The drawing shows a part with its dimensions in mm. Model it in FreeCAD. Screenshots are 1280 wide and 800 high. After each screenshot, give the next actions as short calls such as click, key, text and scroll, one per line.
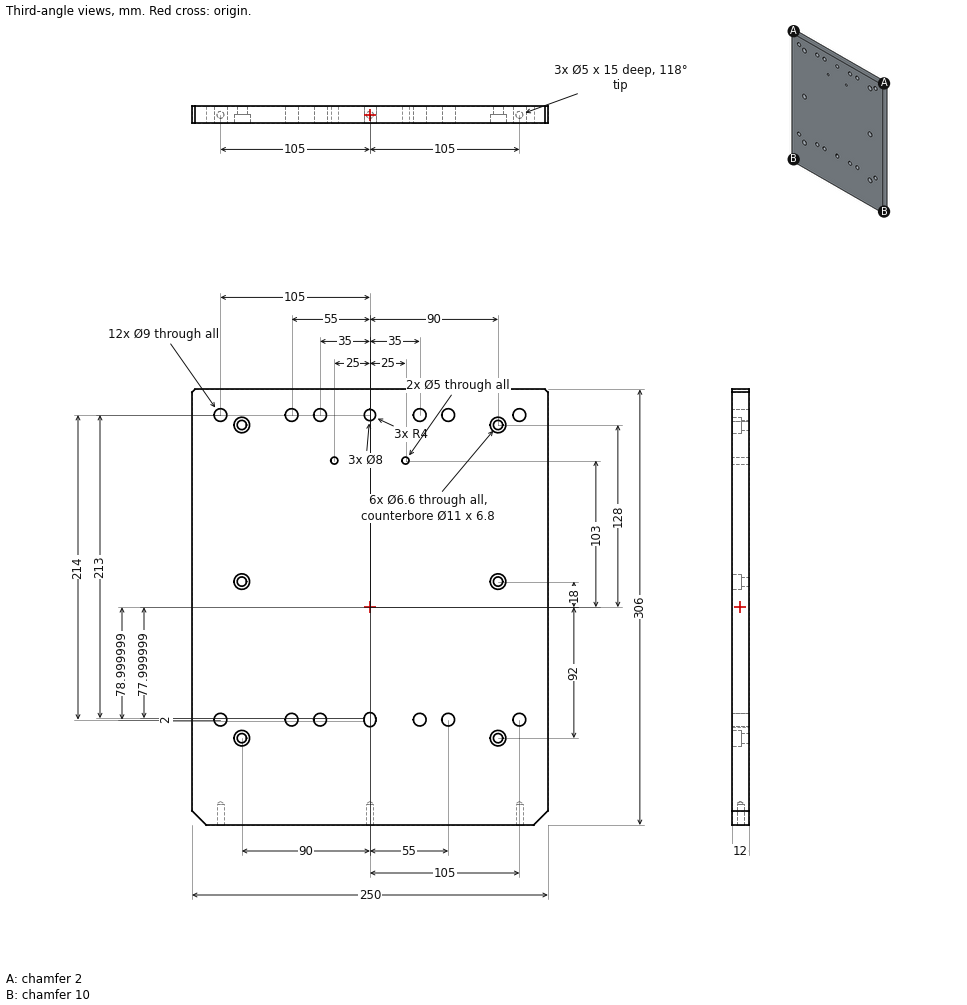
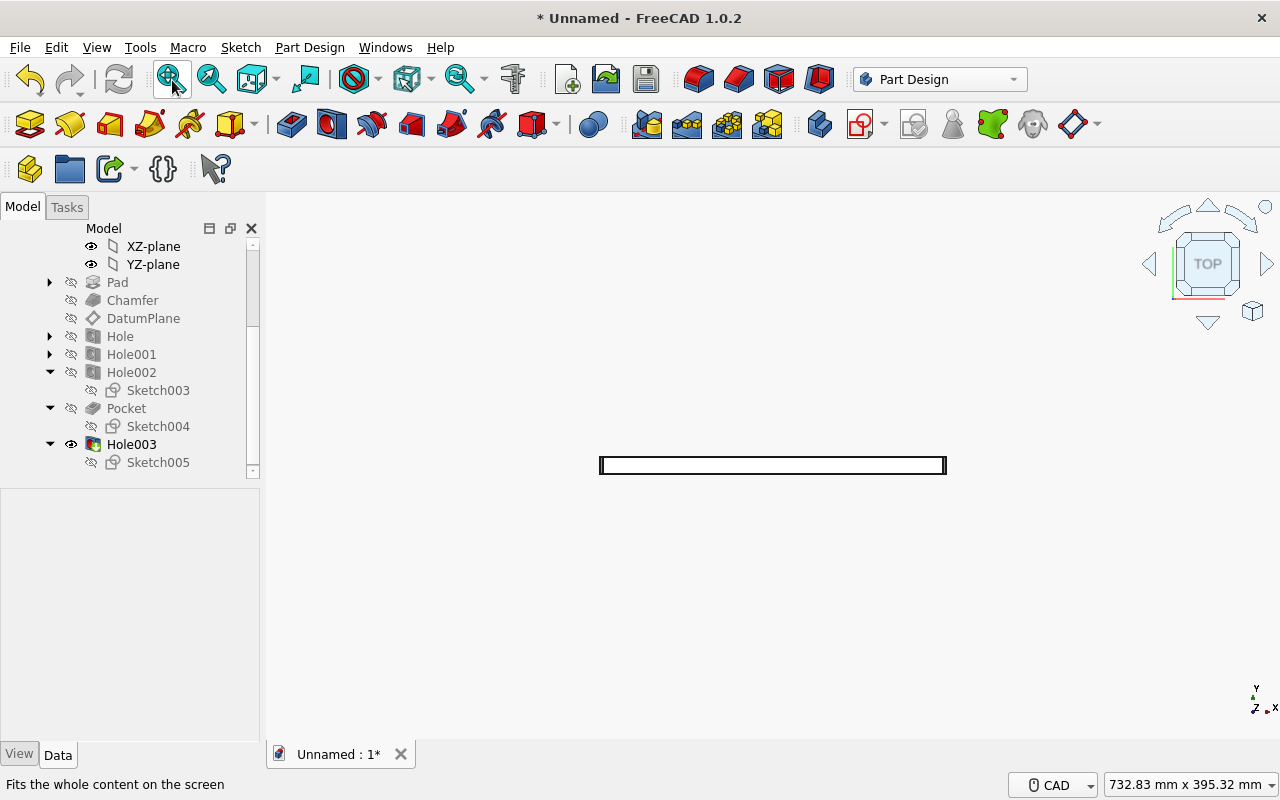
click(172, 80)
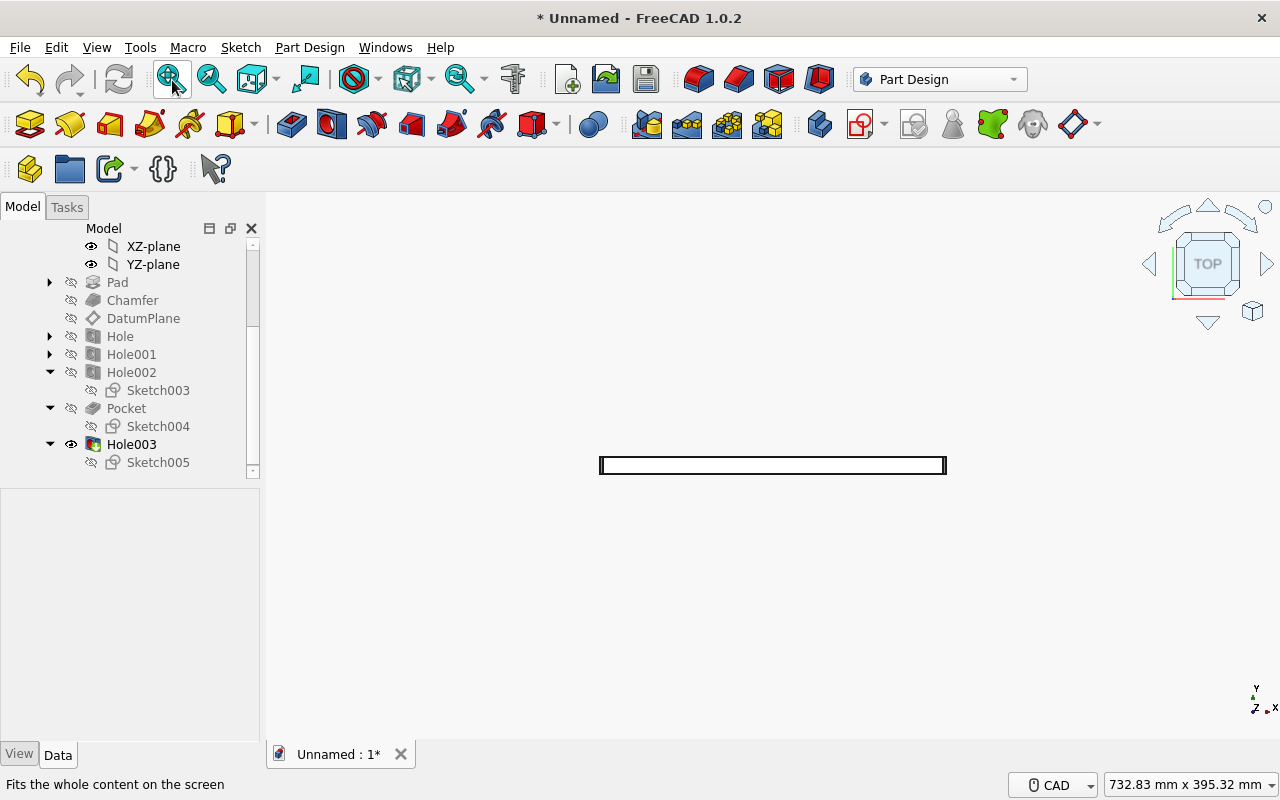
scroll(600, 464, up, 5)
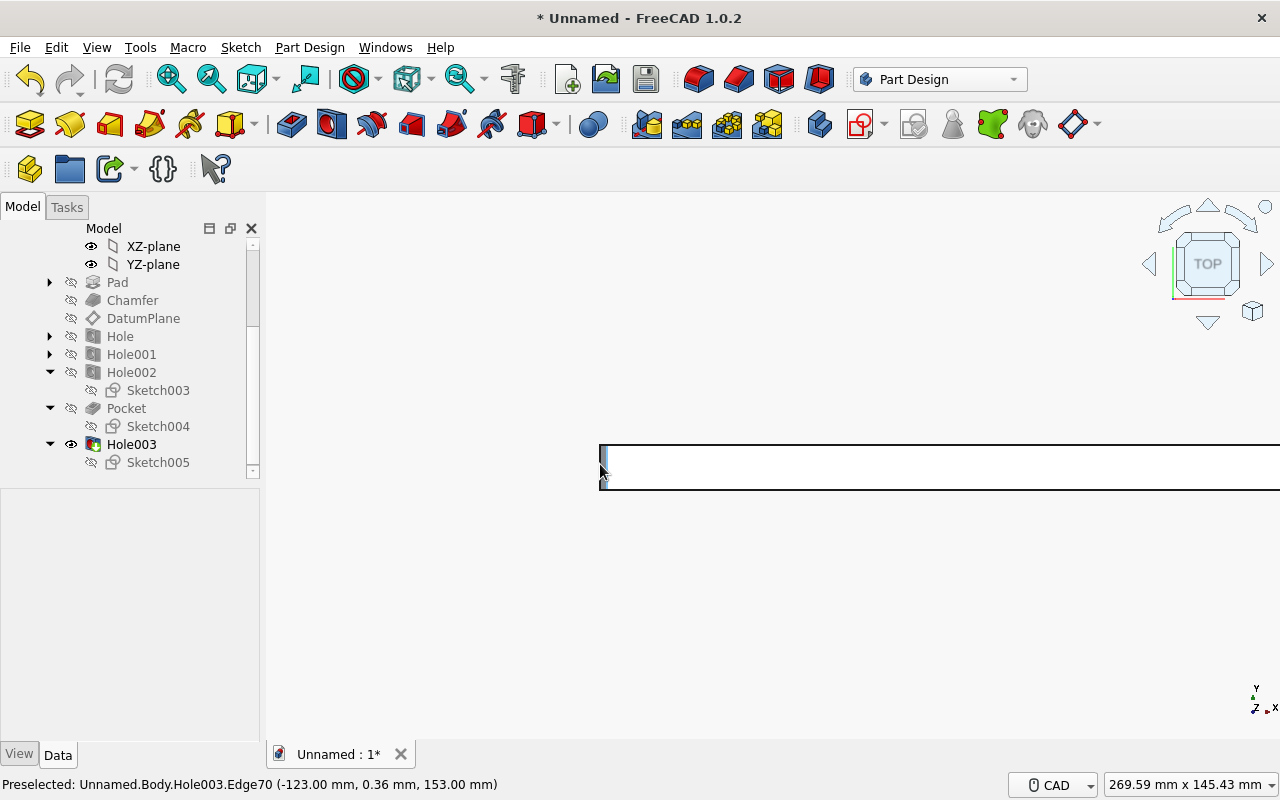
click(172, 80)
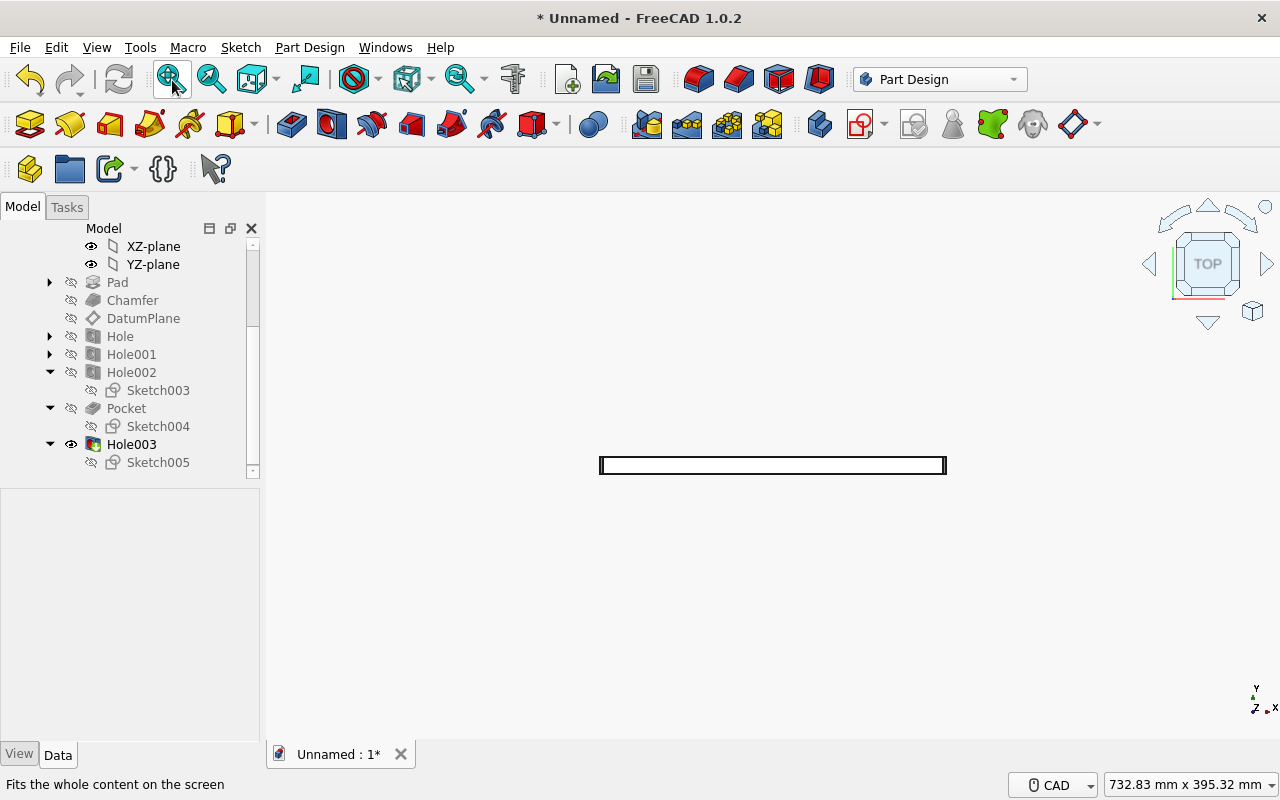
key(1)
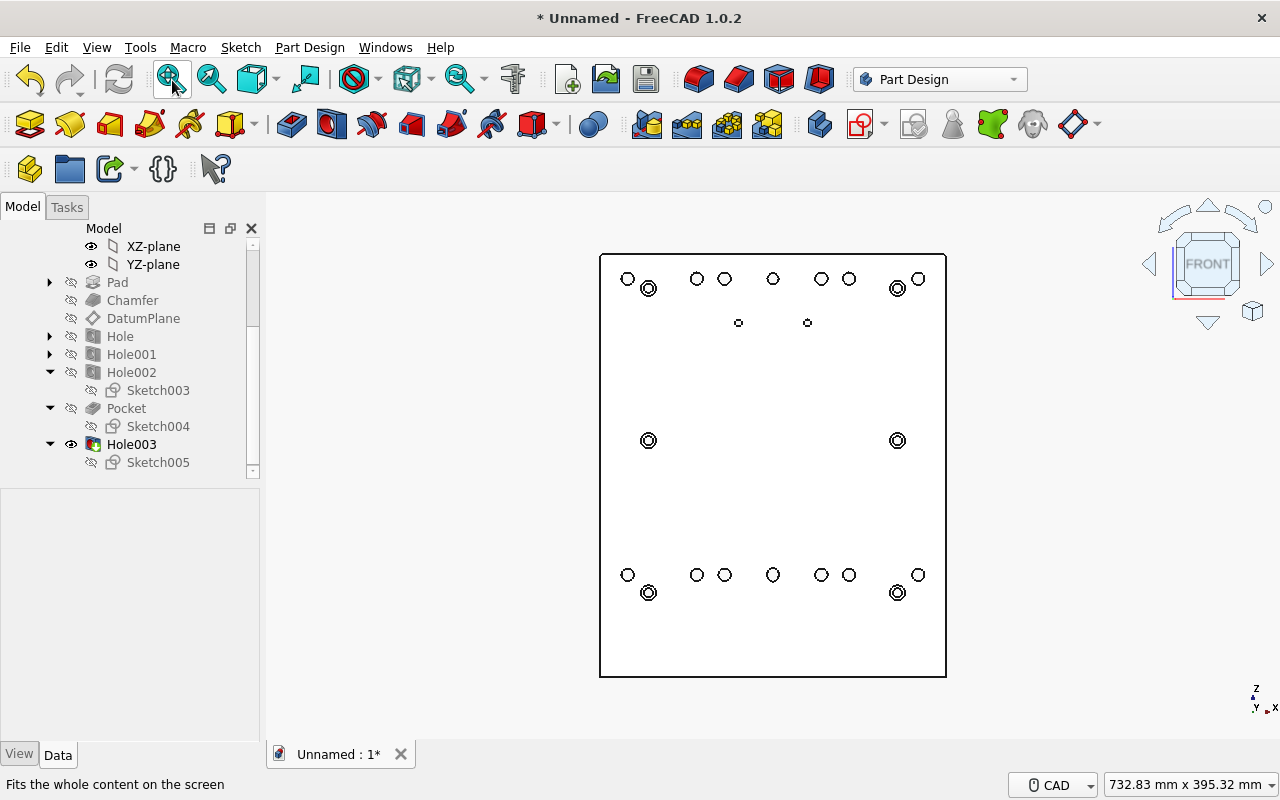
scroll(600, 676, up, 5)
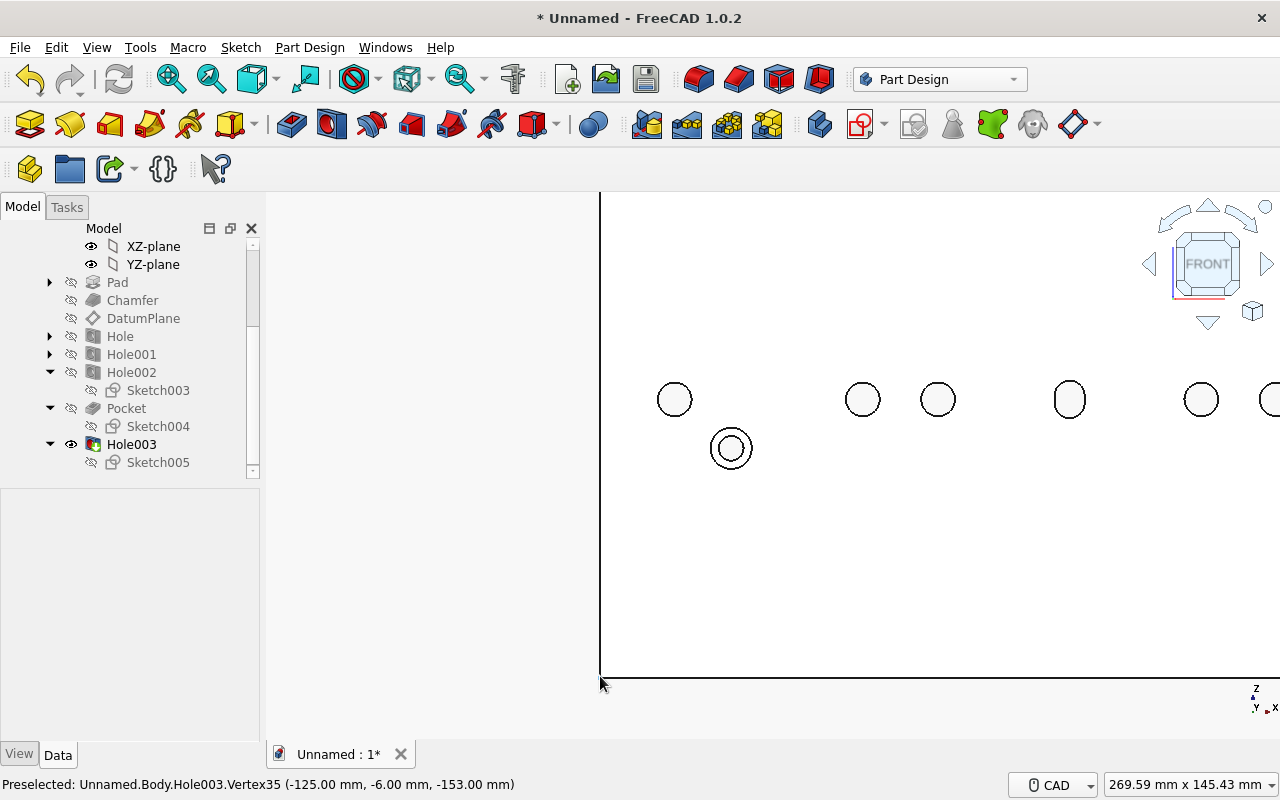
key(v)
key(f)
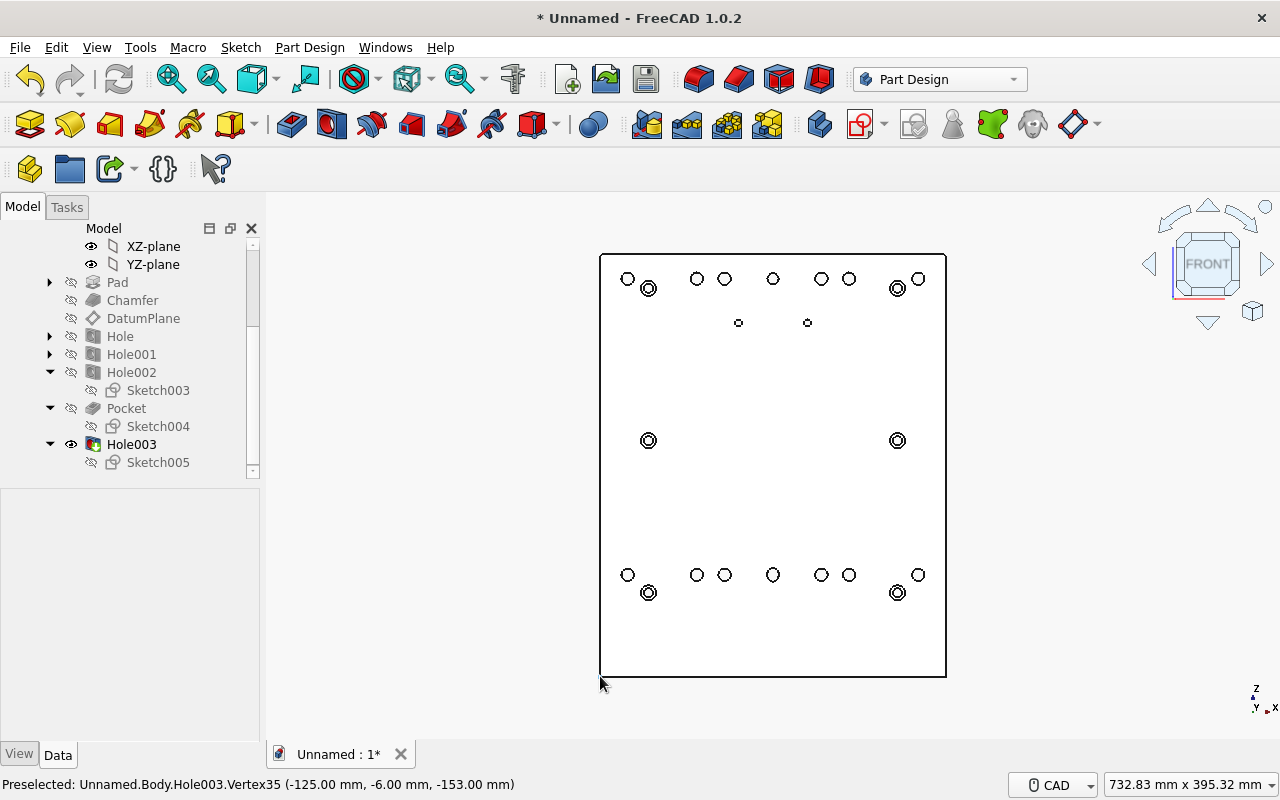
key(3)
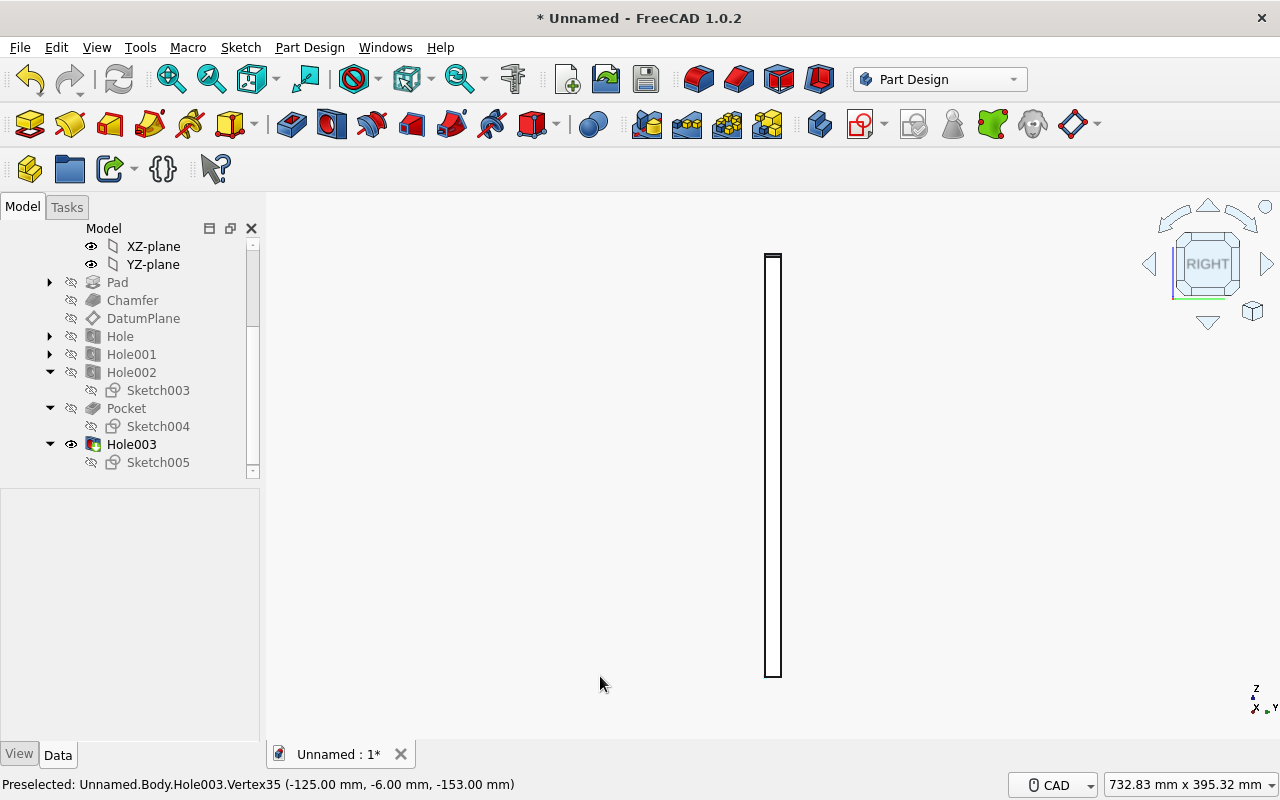
click(773, 676)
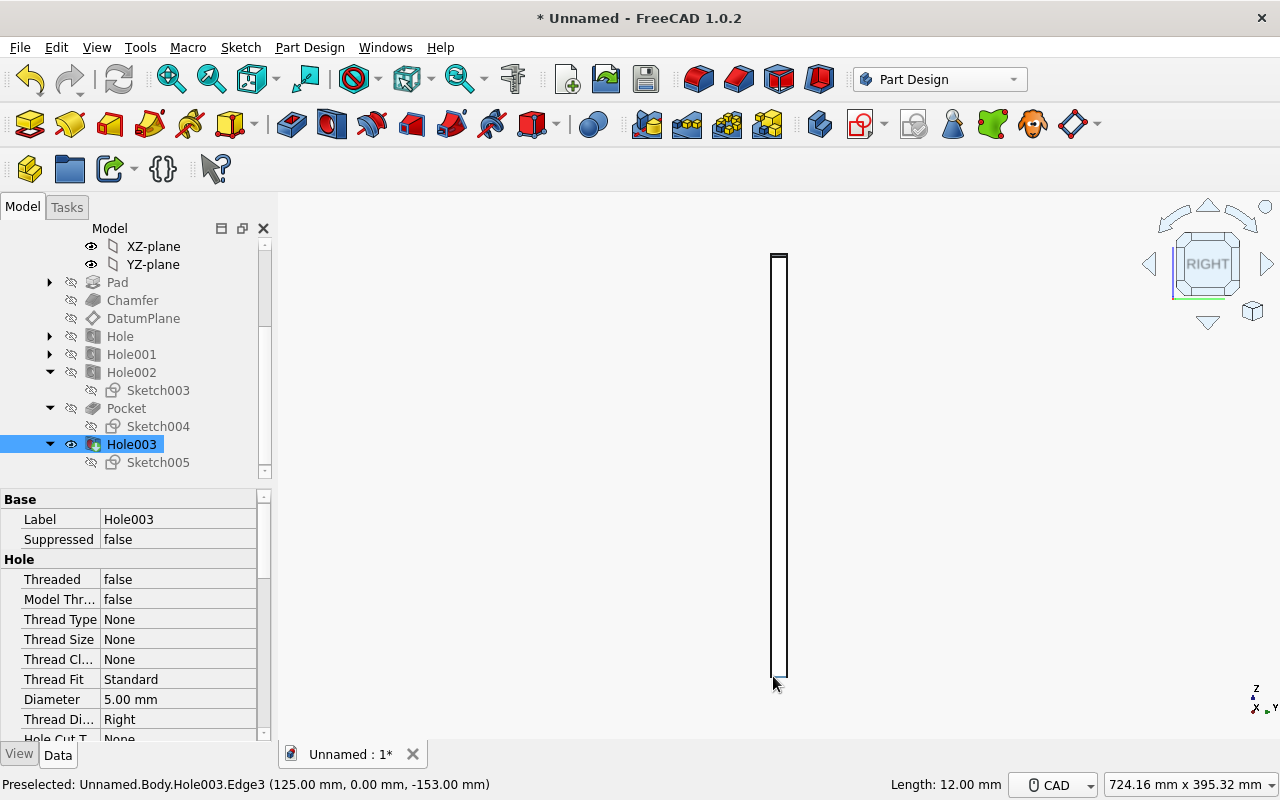
scroll(779, 676, up, 5)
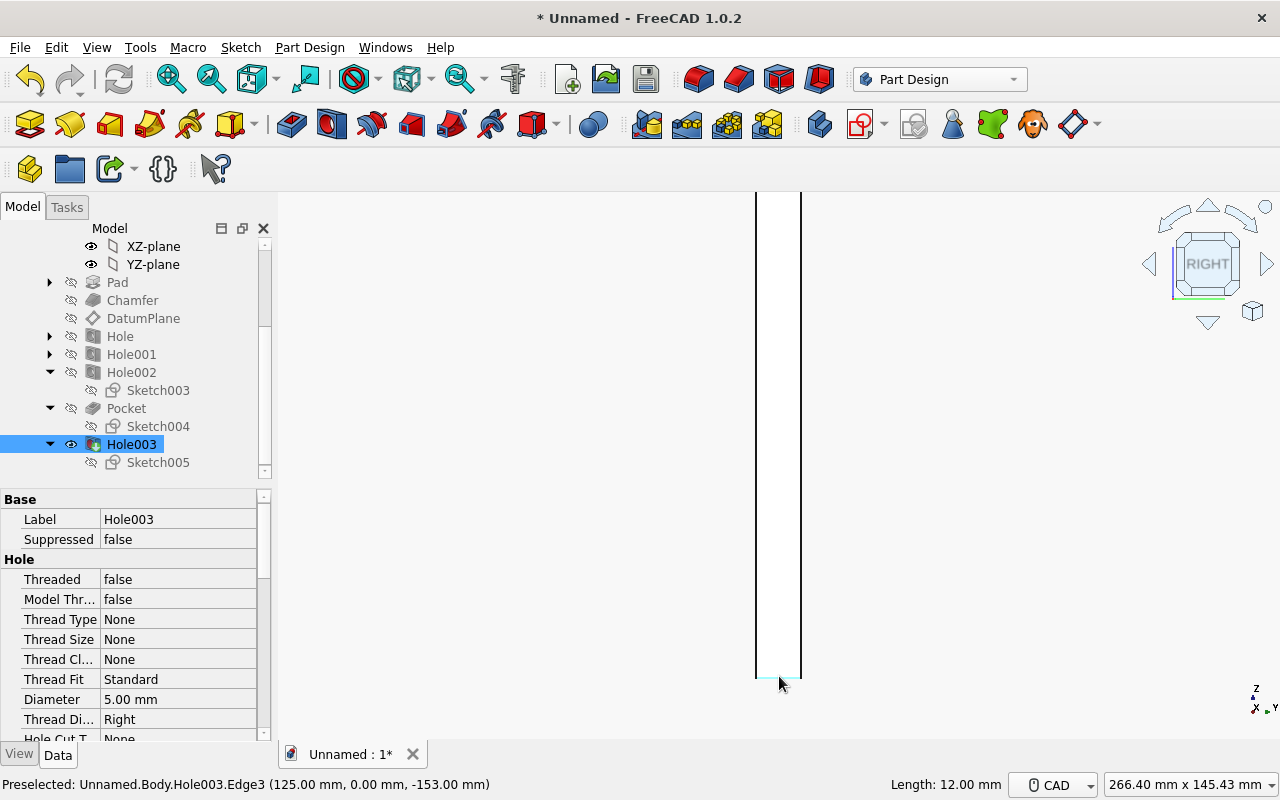
key(v)
key(f)